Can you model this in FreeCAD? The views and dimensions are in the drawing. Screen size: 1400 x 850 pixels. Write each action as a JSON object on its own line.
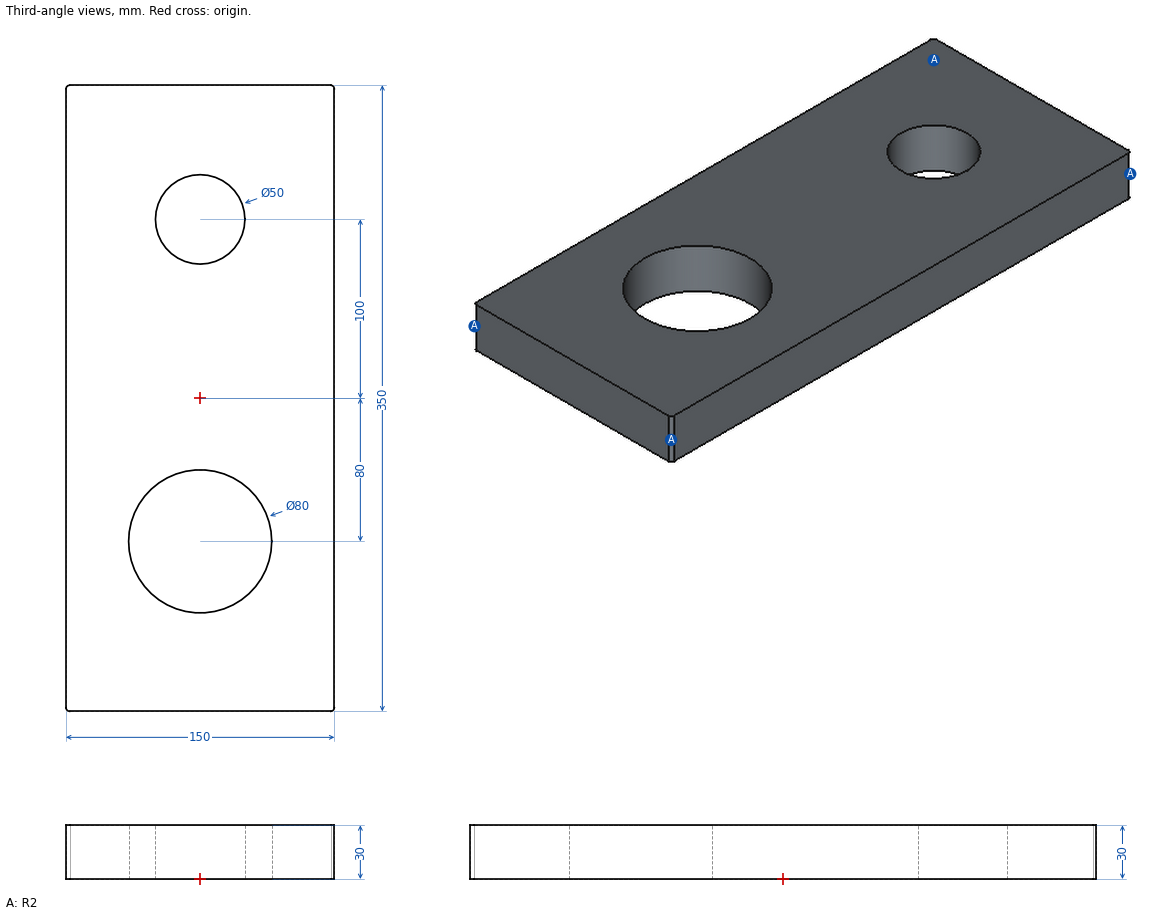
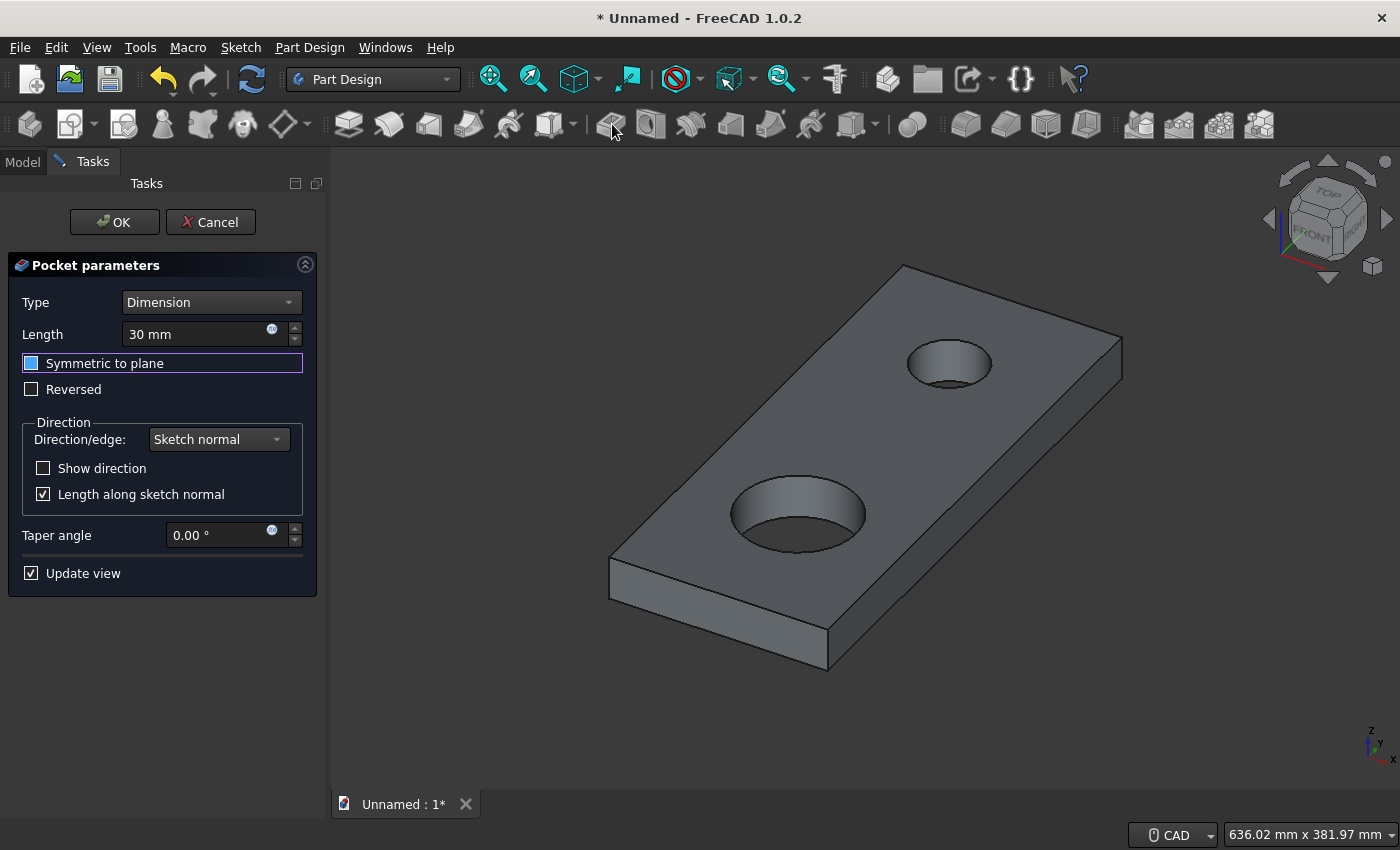
{"action": "left_click", "coordinate": [115, 222]}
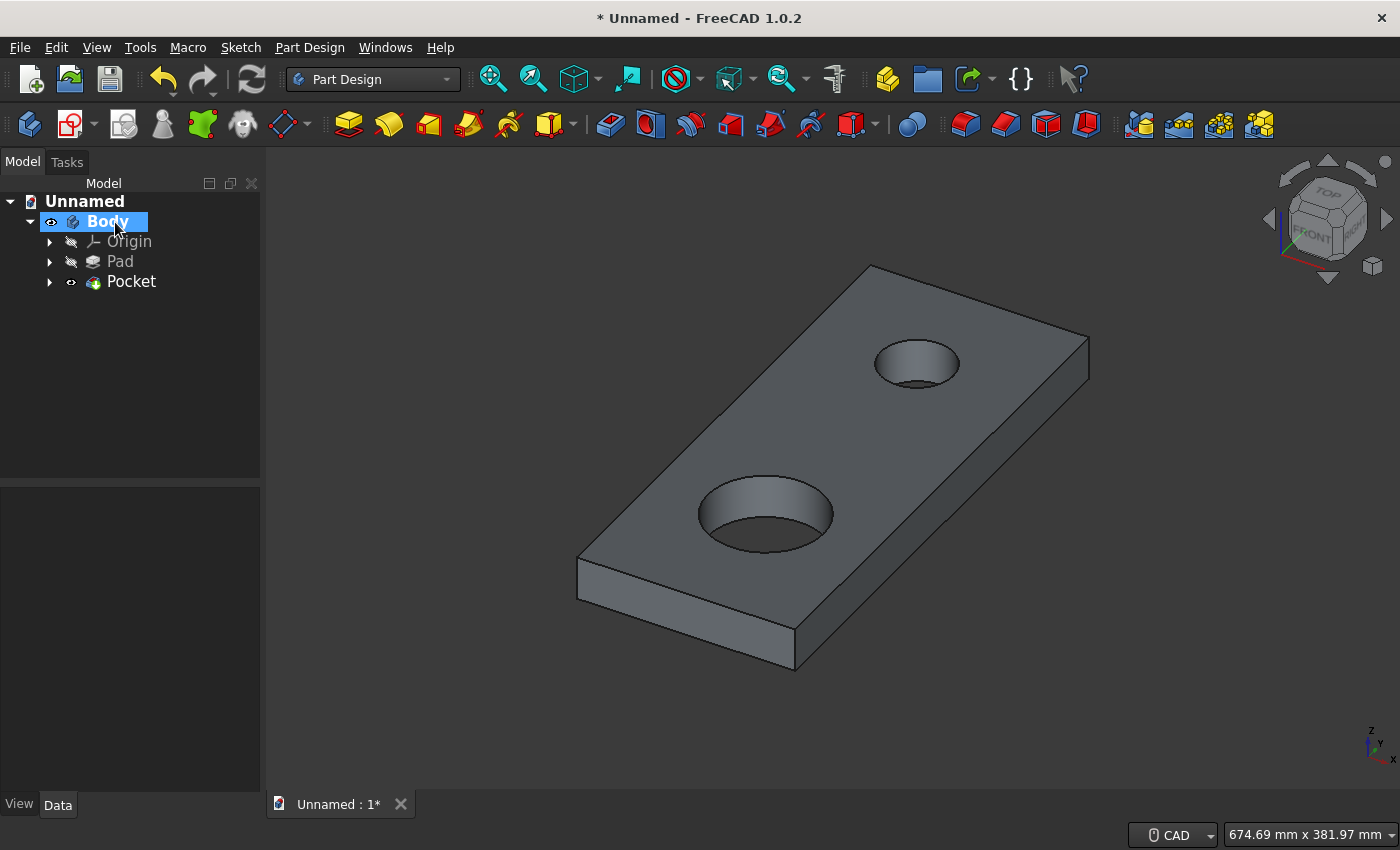
{"action": "left_click", "coordinate": [795, 649]}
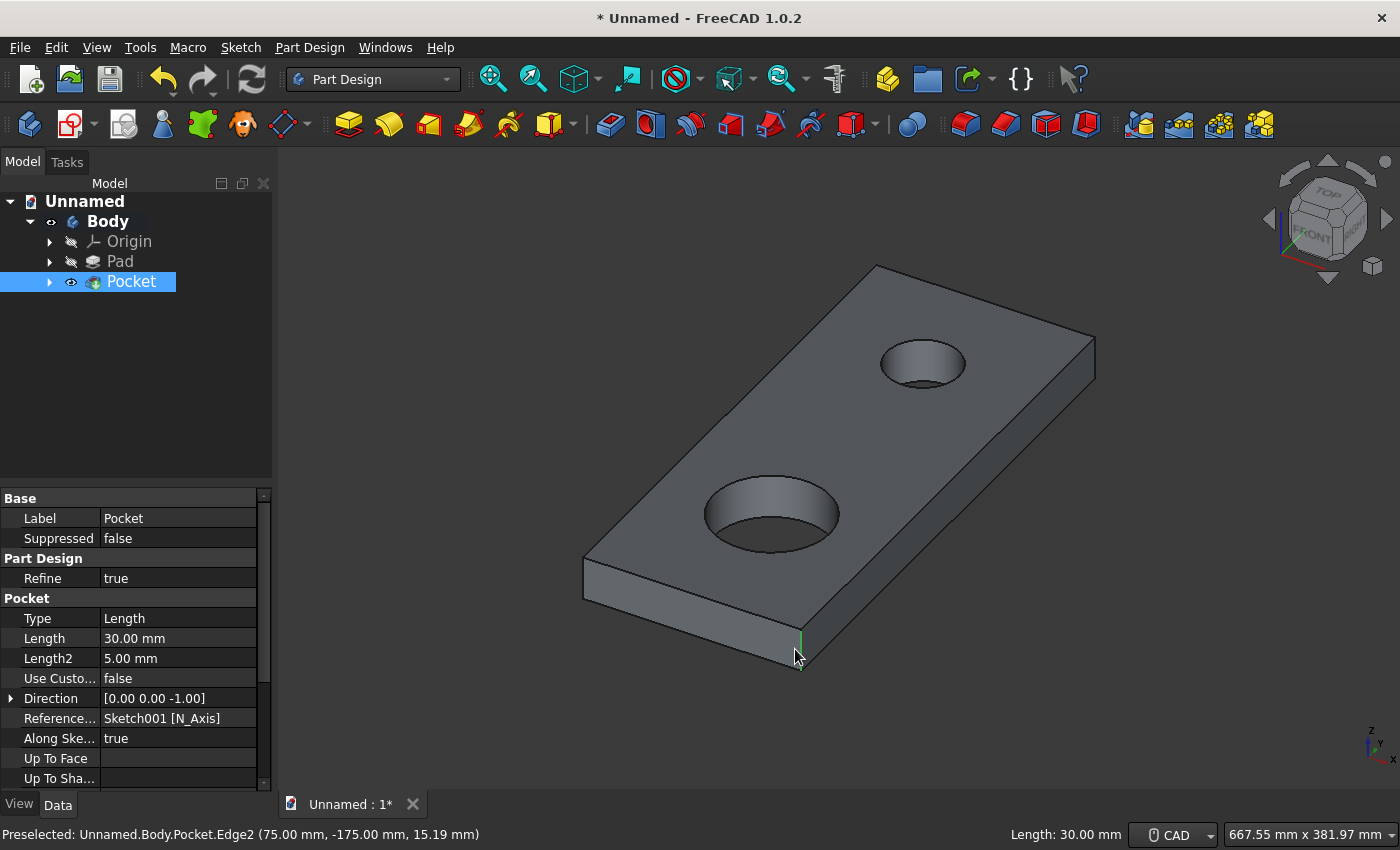
{"action": "key", "text": "0"}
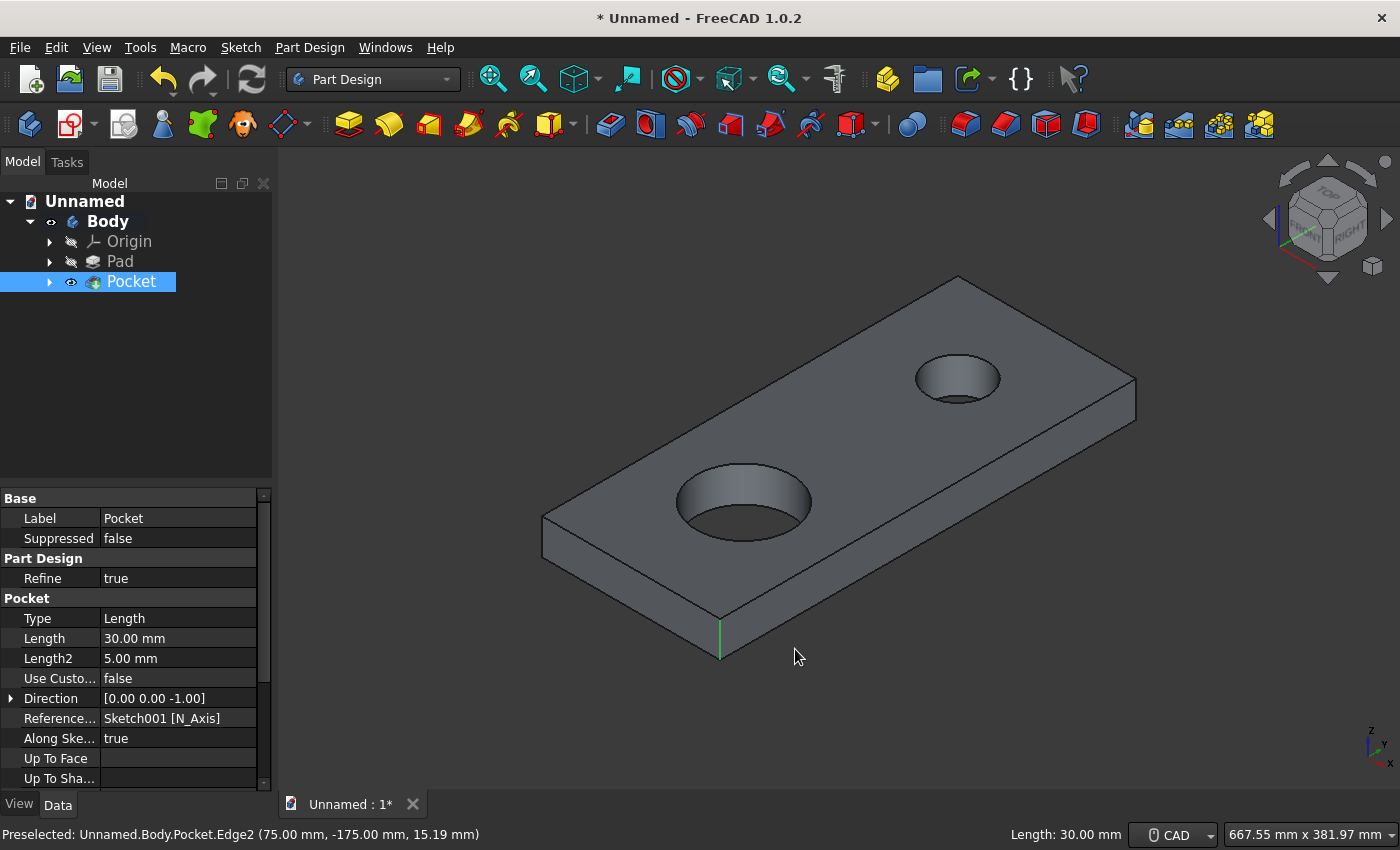
{"action": "key", "text": "2"}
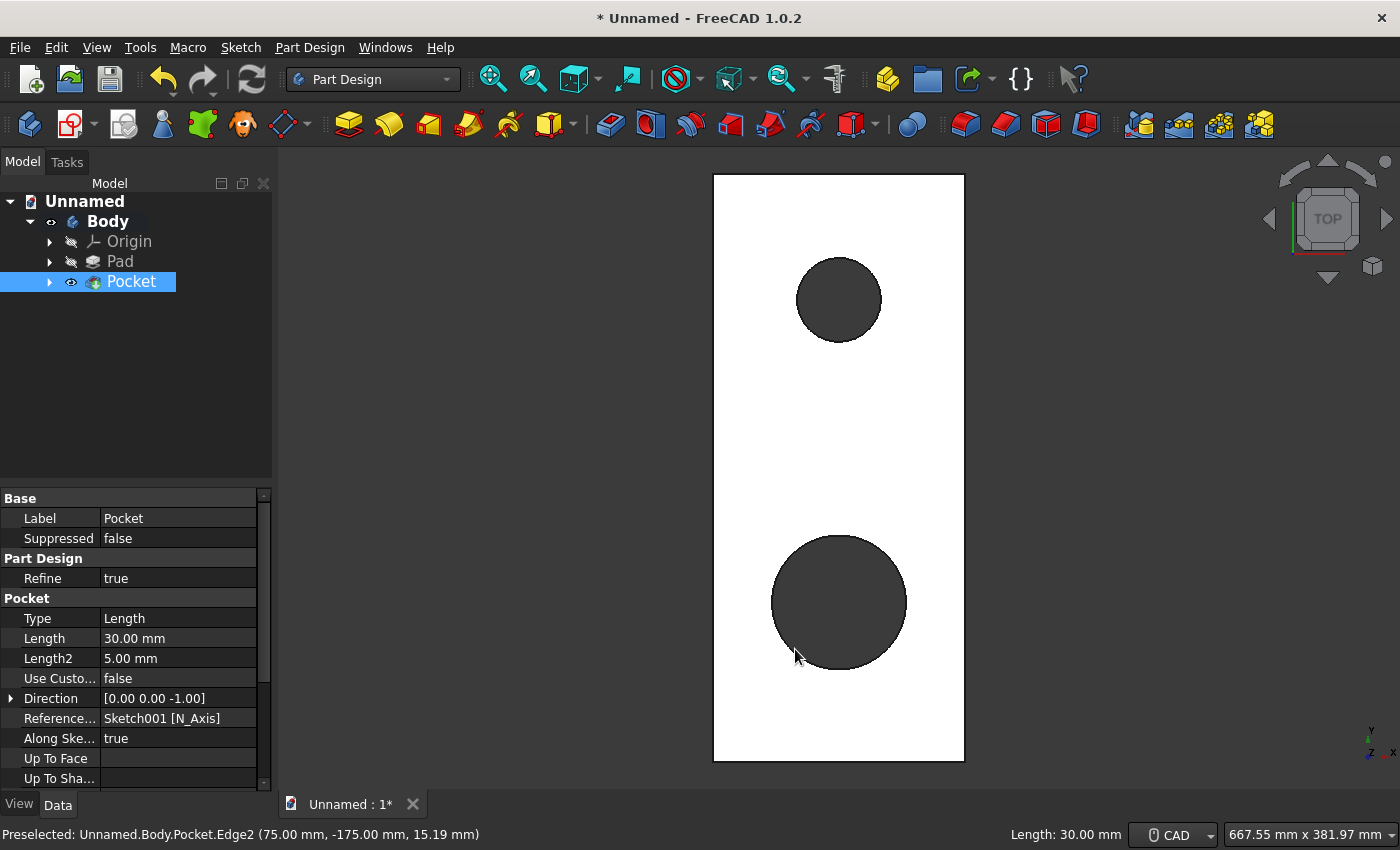
{"action": "key", "text": "1"}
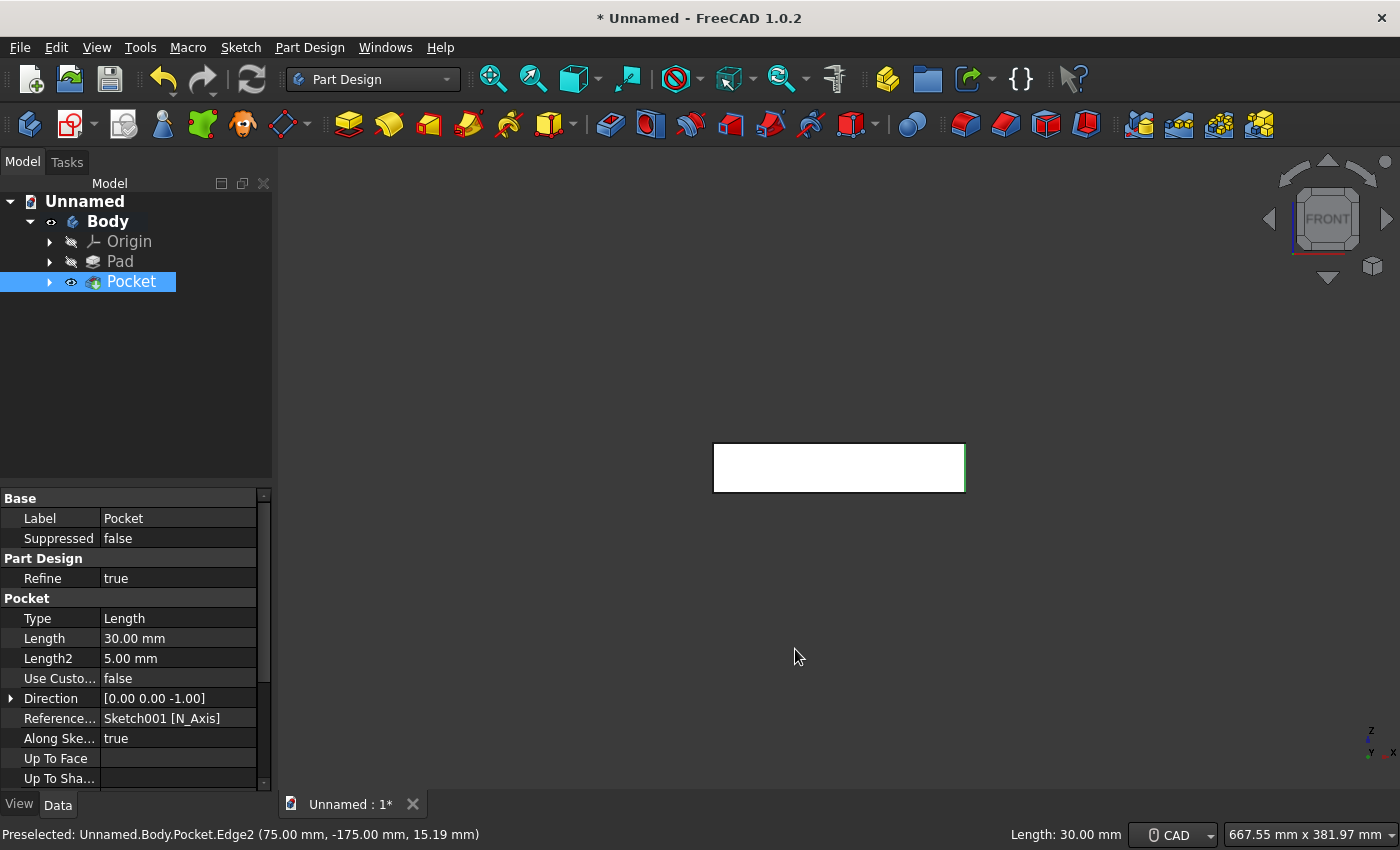
{"action": "left_click", "coordinate": [494, 80]}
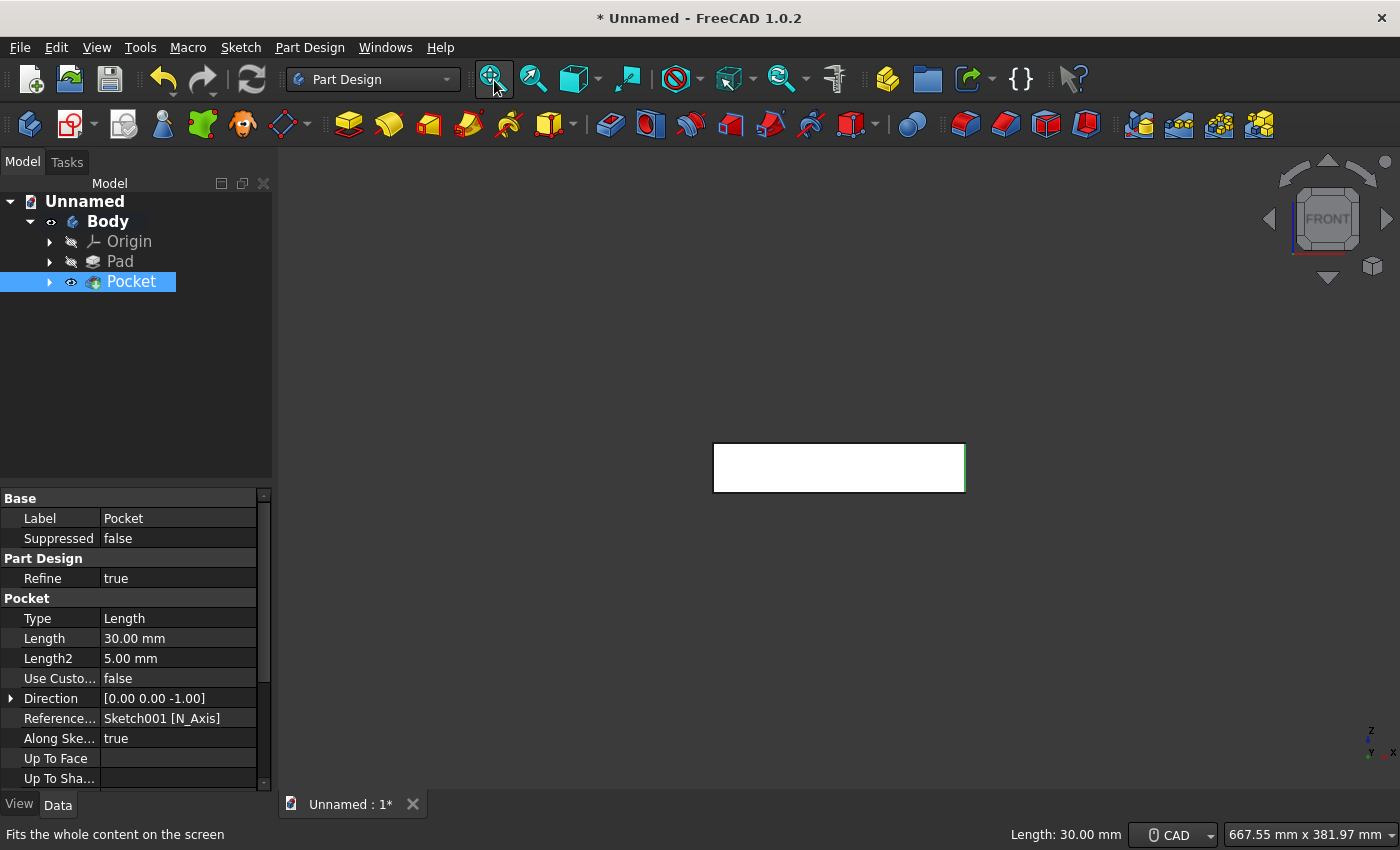
{"action": "left_click", "coordinate": [713, 467], "text": "ctrl"}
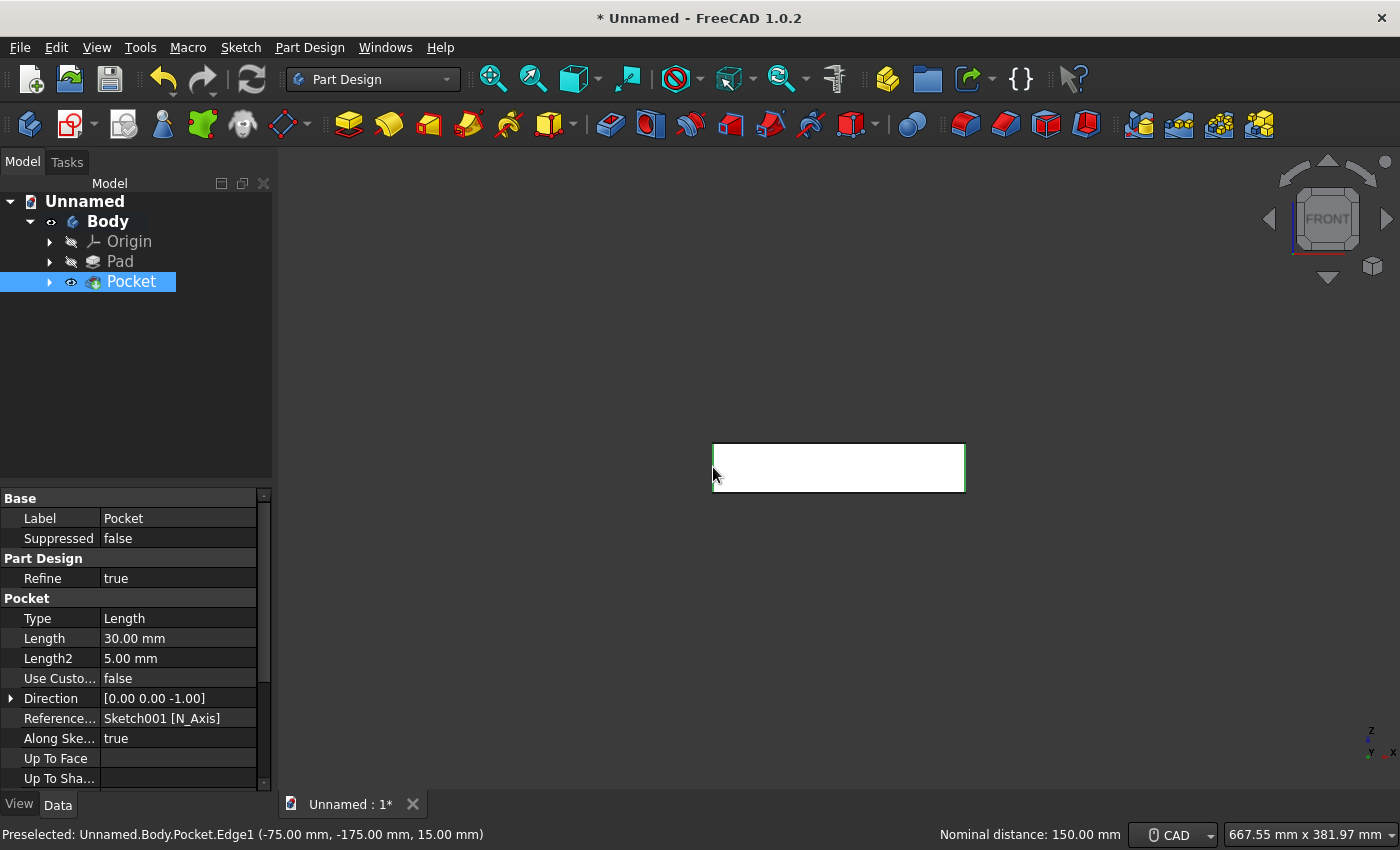
{"action": "key", "text": "3"}